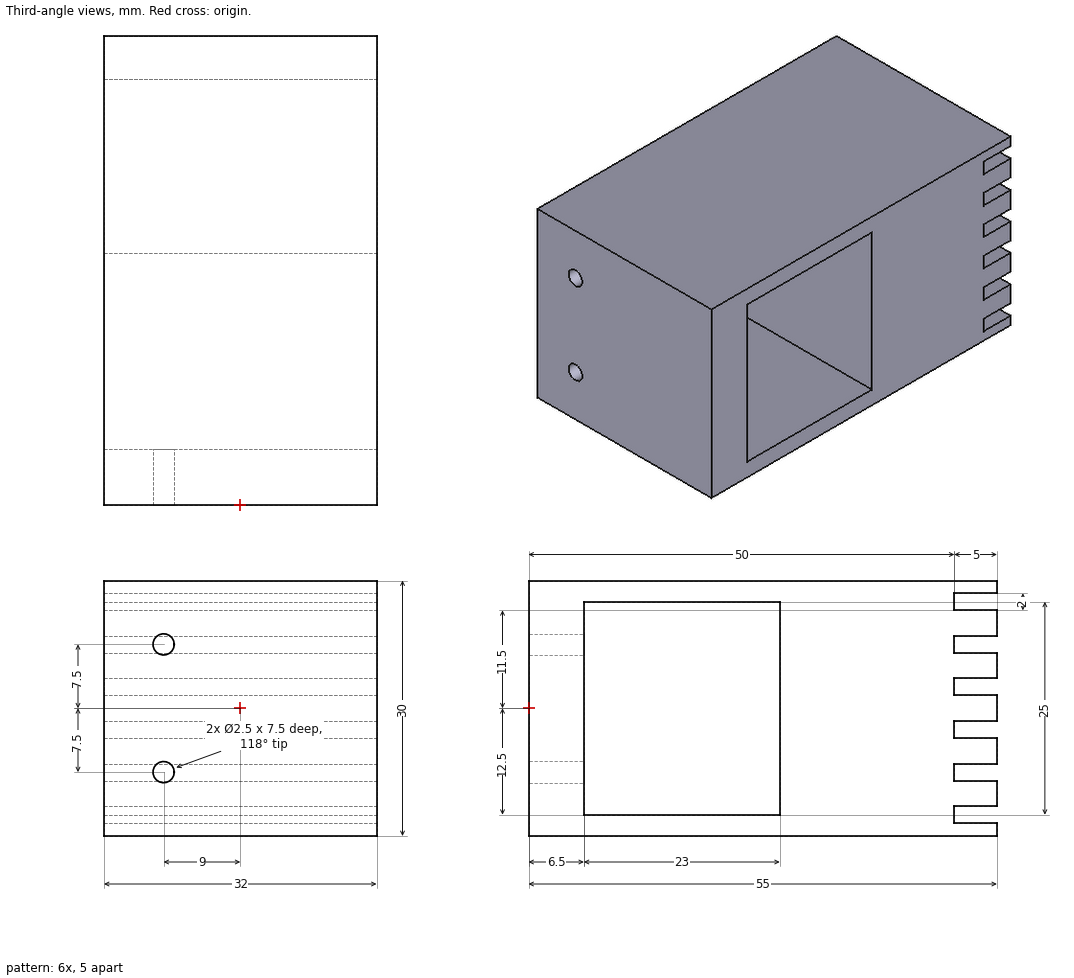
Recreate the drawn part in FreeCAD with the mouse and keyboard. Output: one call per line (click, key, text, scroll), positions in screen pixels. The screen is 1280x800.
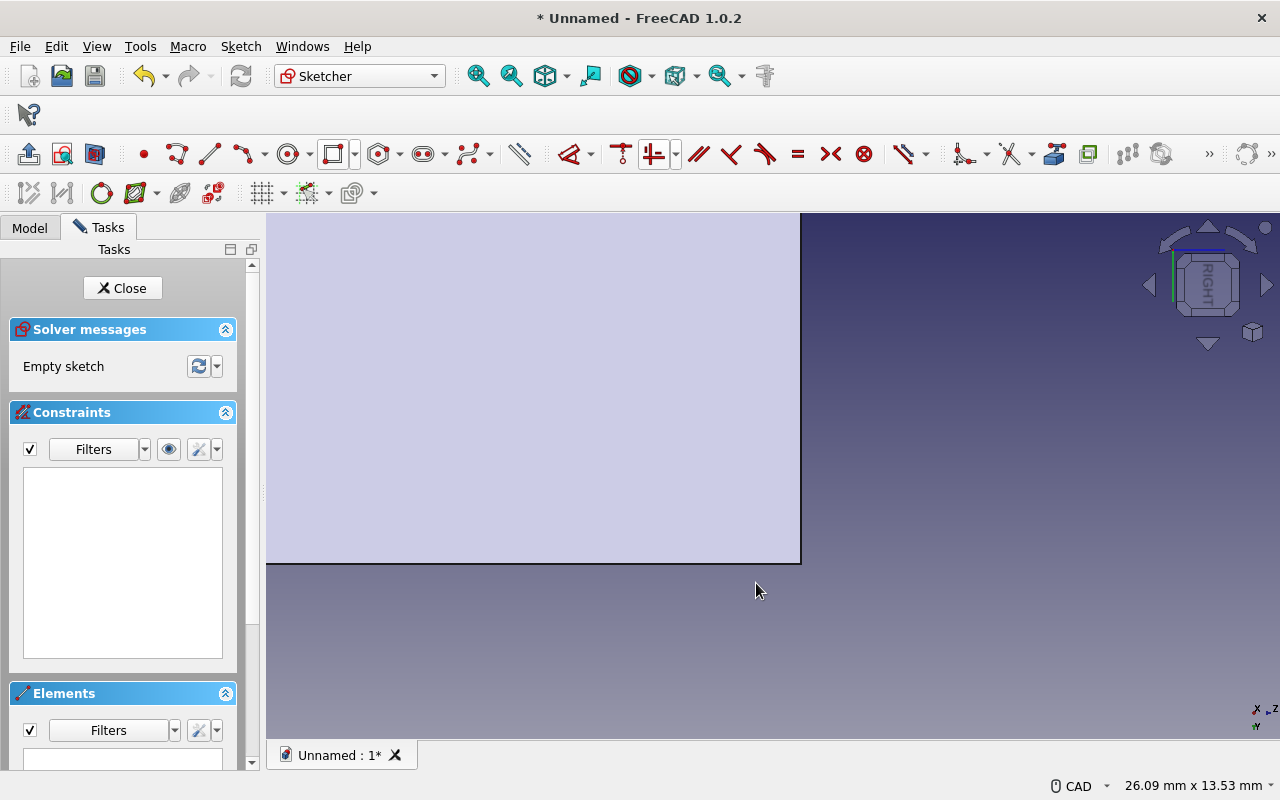
scroll(702, 457, up, 3)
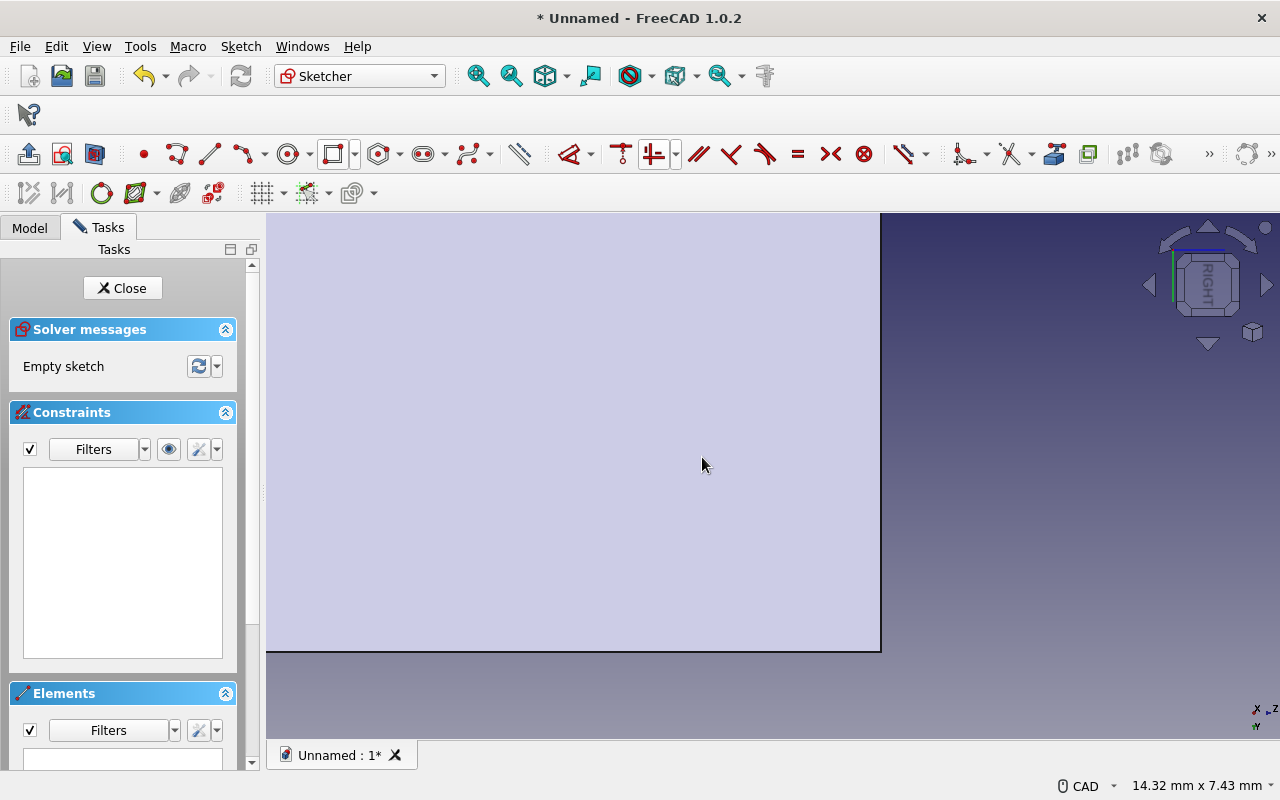
click(332, 154)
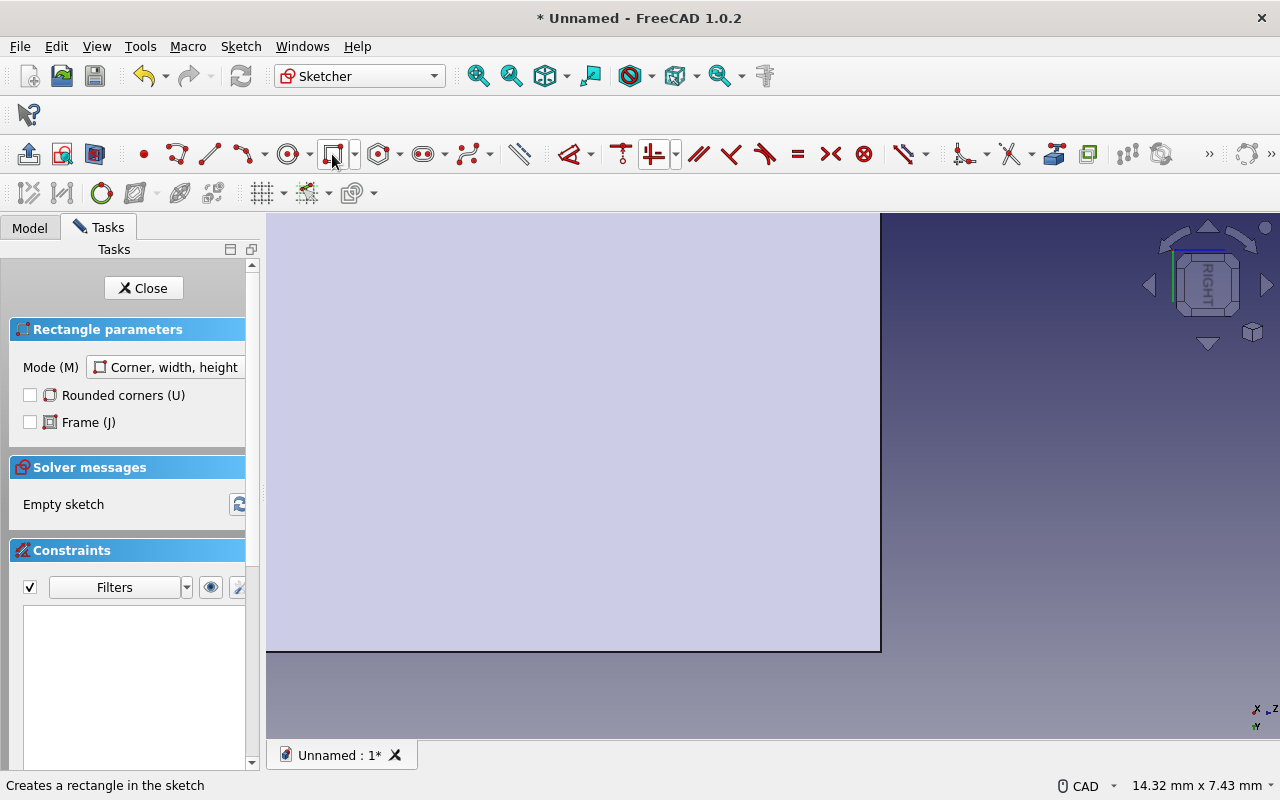
click(634, 298)
click(775, 652)
key(Escape)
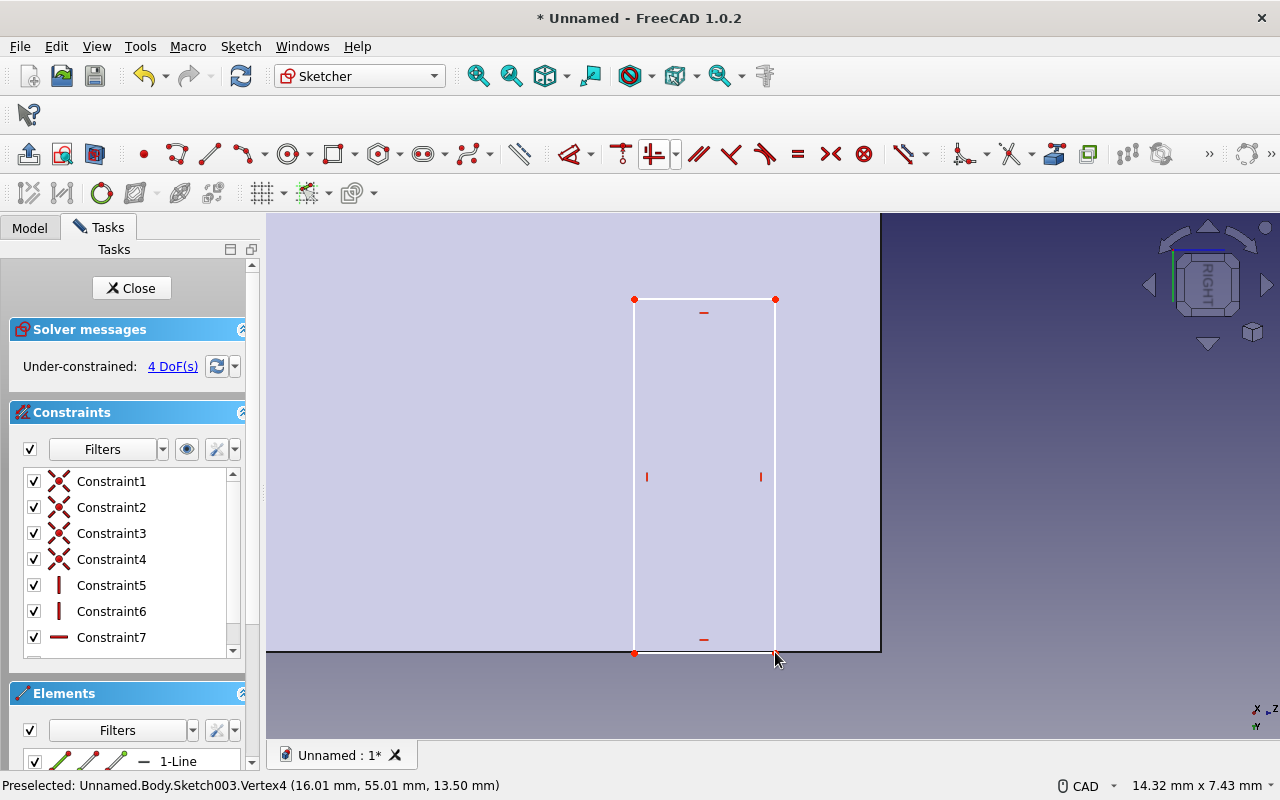
click(568, 154)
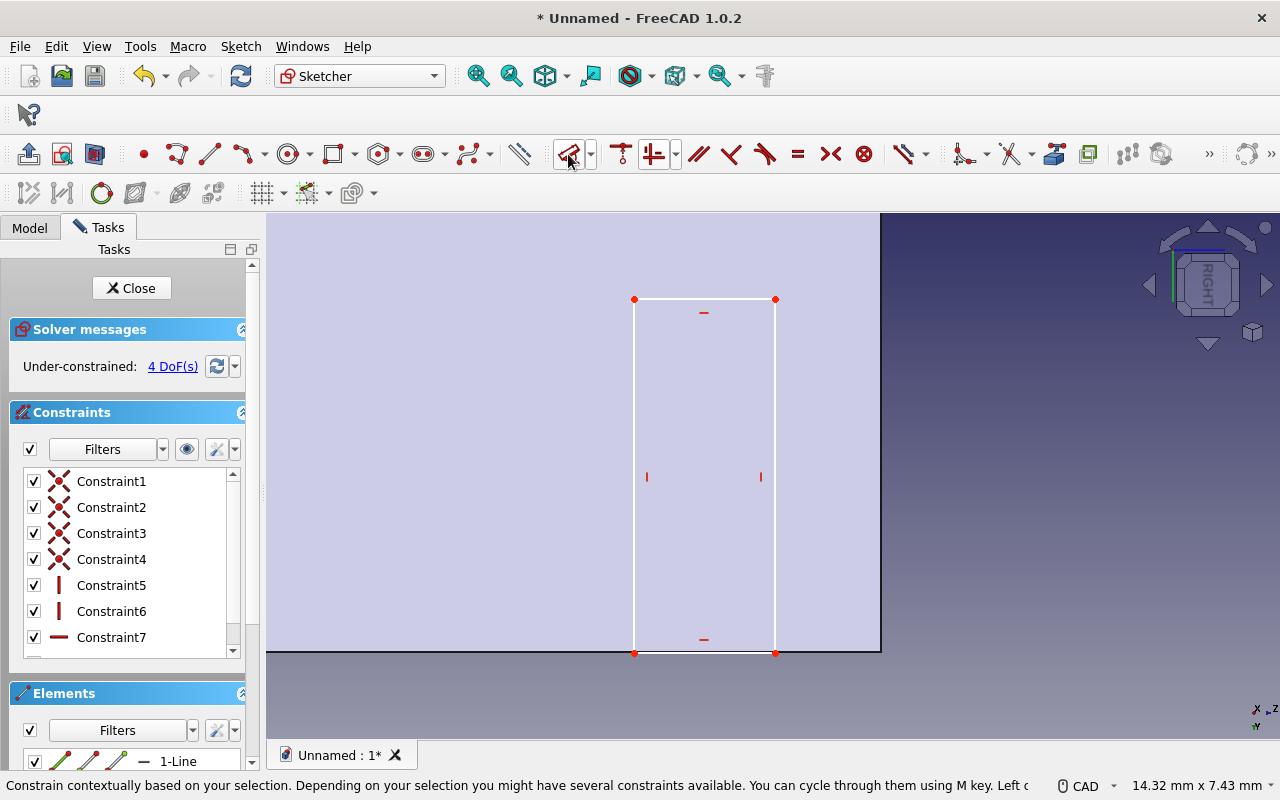
click(634, 405)
click(600, 476)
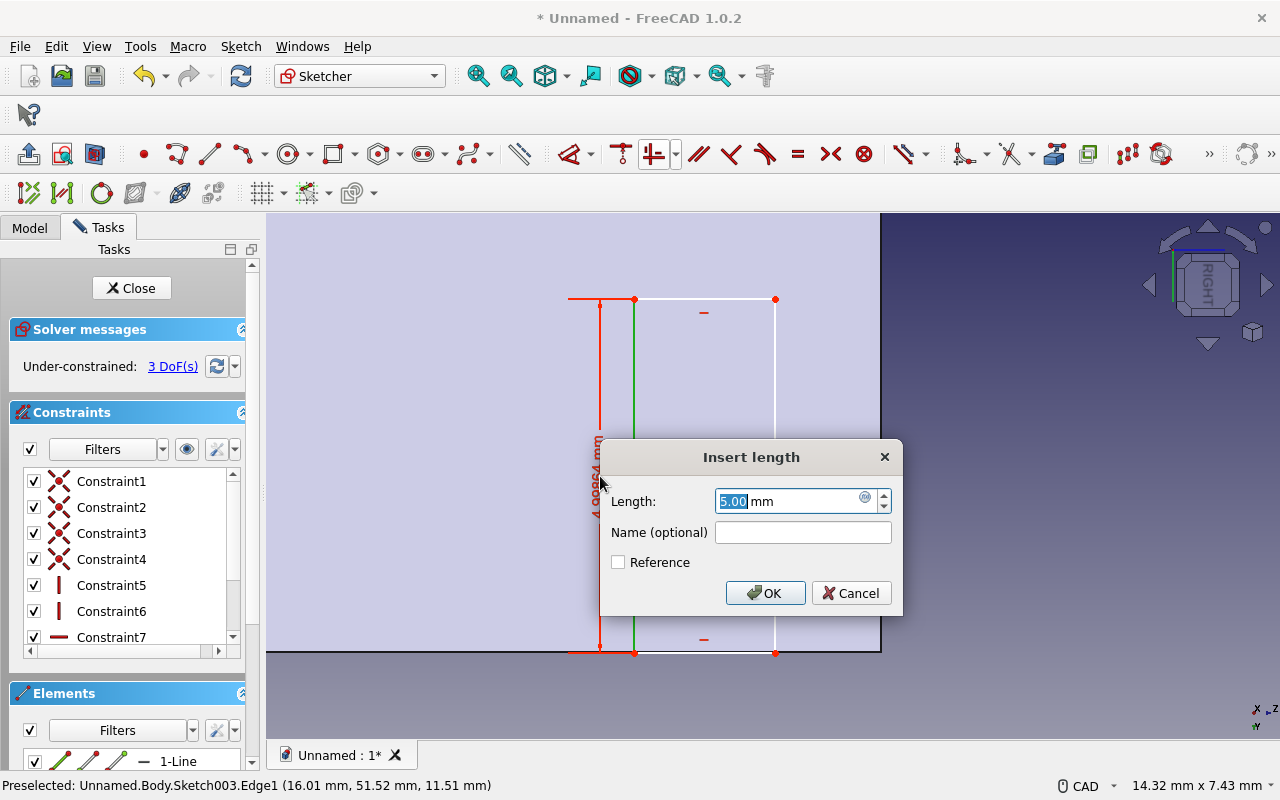
text(5)
key(Return)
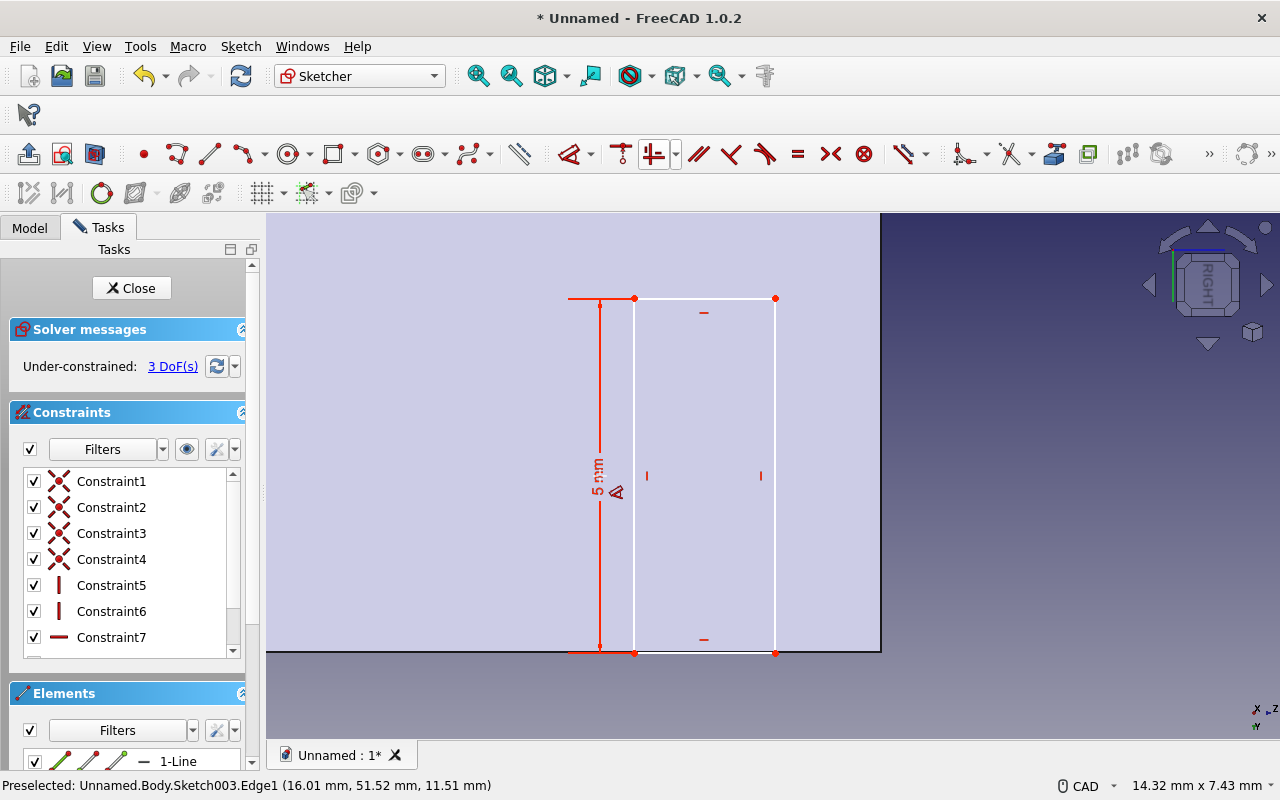
click(676, 653)
click(704, 687)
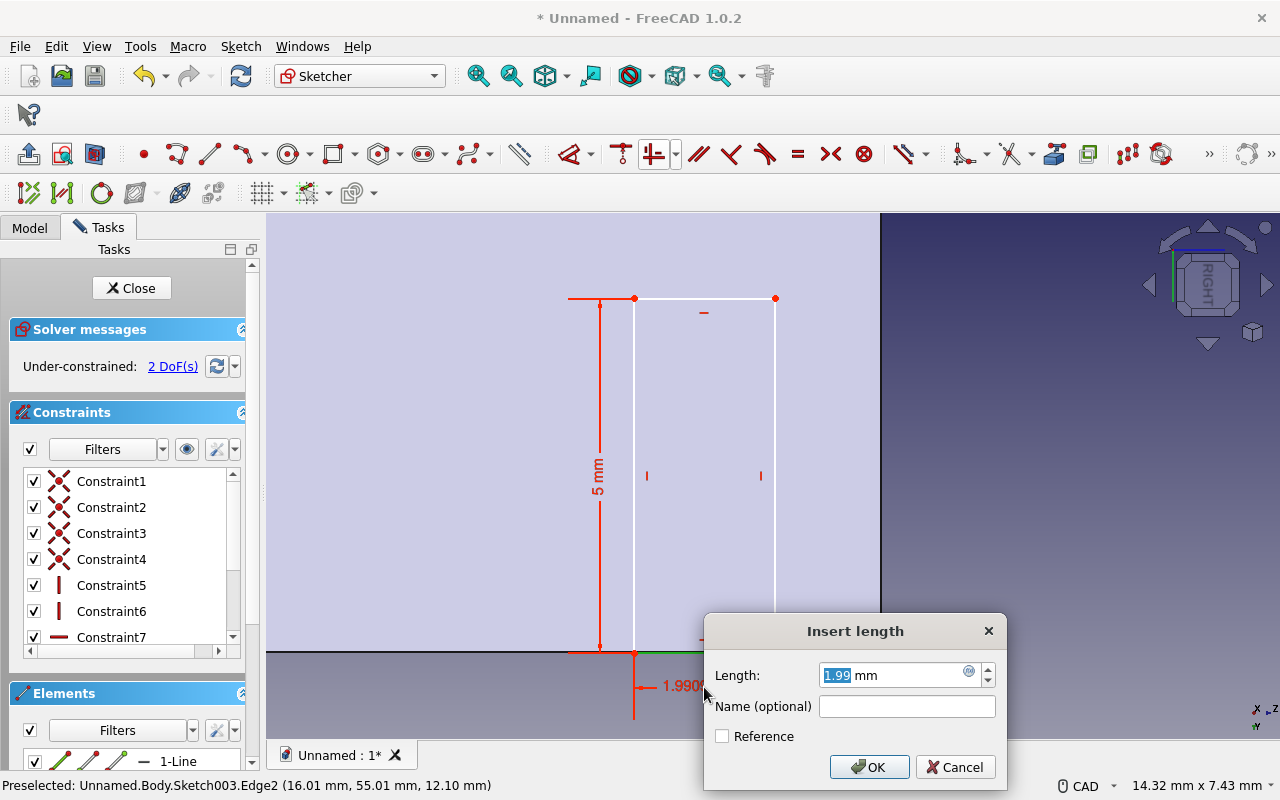
text(2)
key(Return)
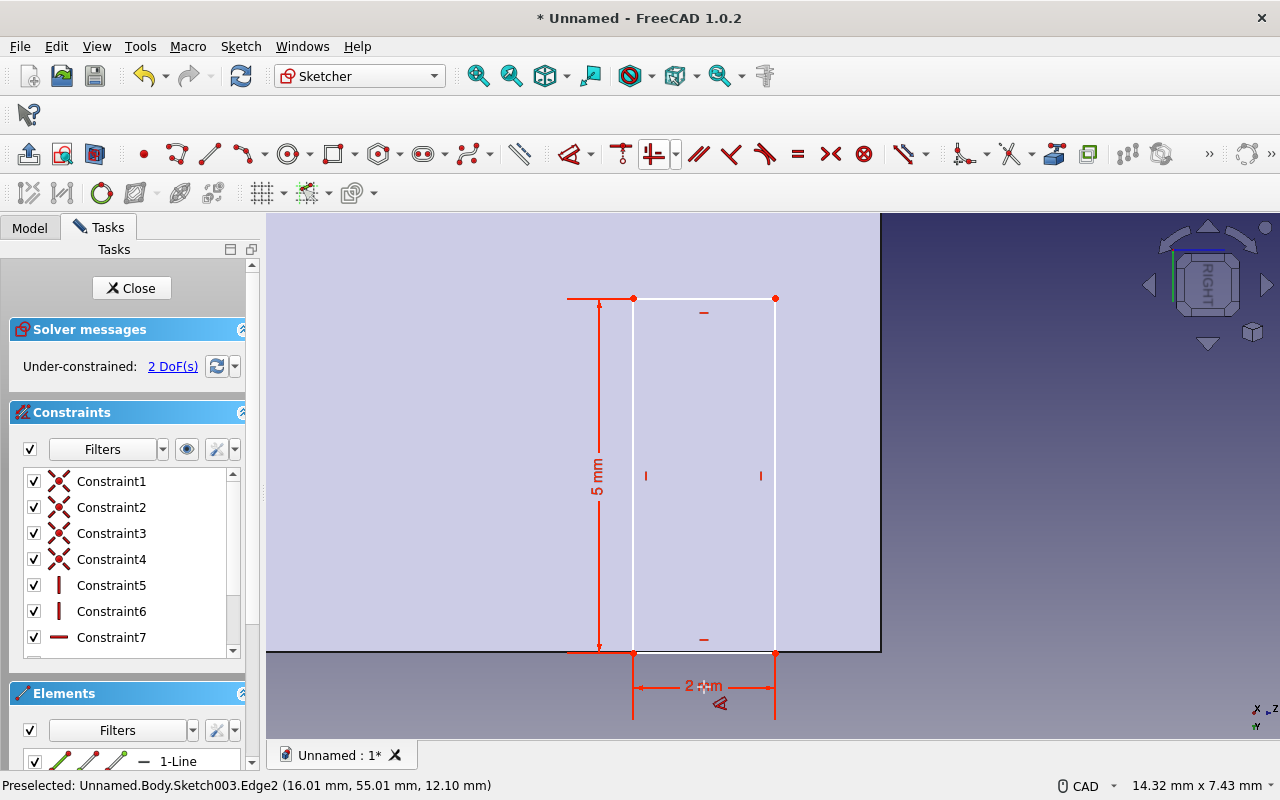
click(633, 299)
click(667, 270)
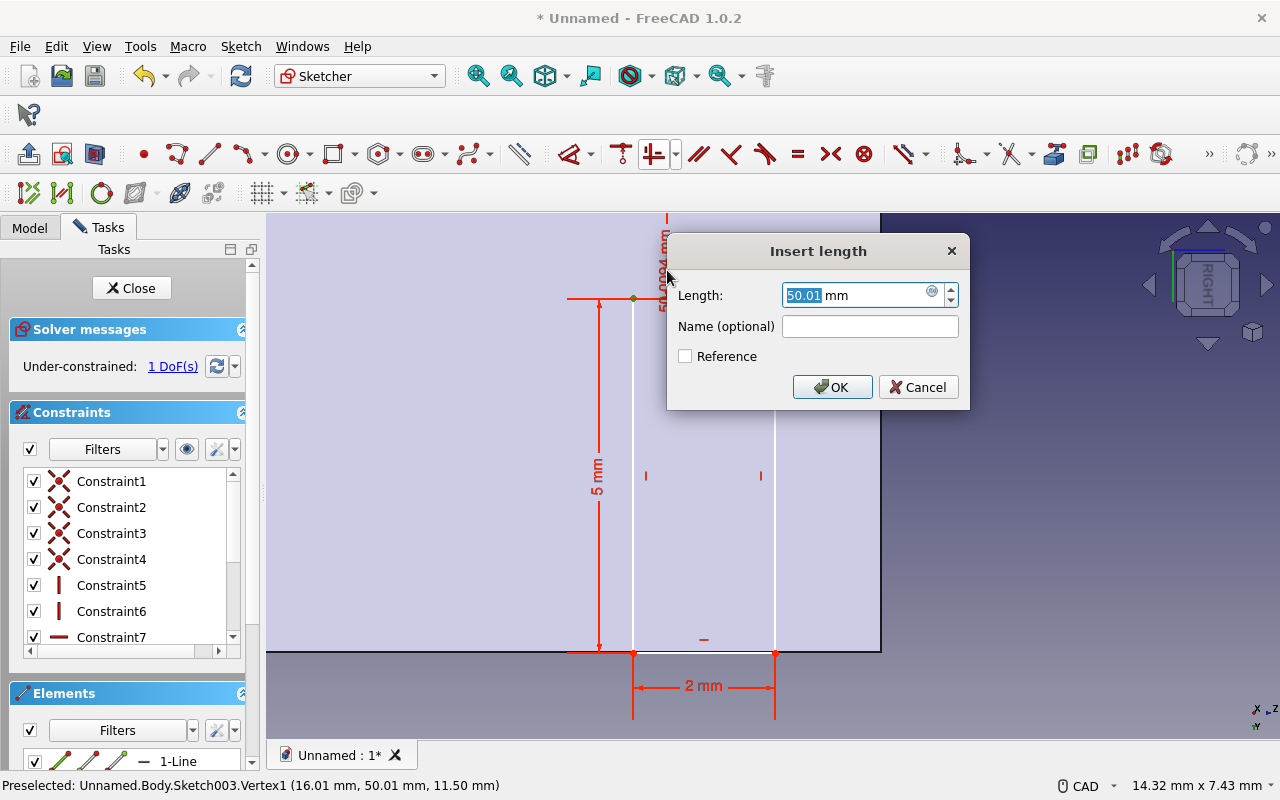
text(50)
key(Return)